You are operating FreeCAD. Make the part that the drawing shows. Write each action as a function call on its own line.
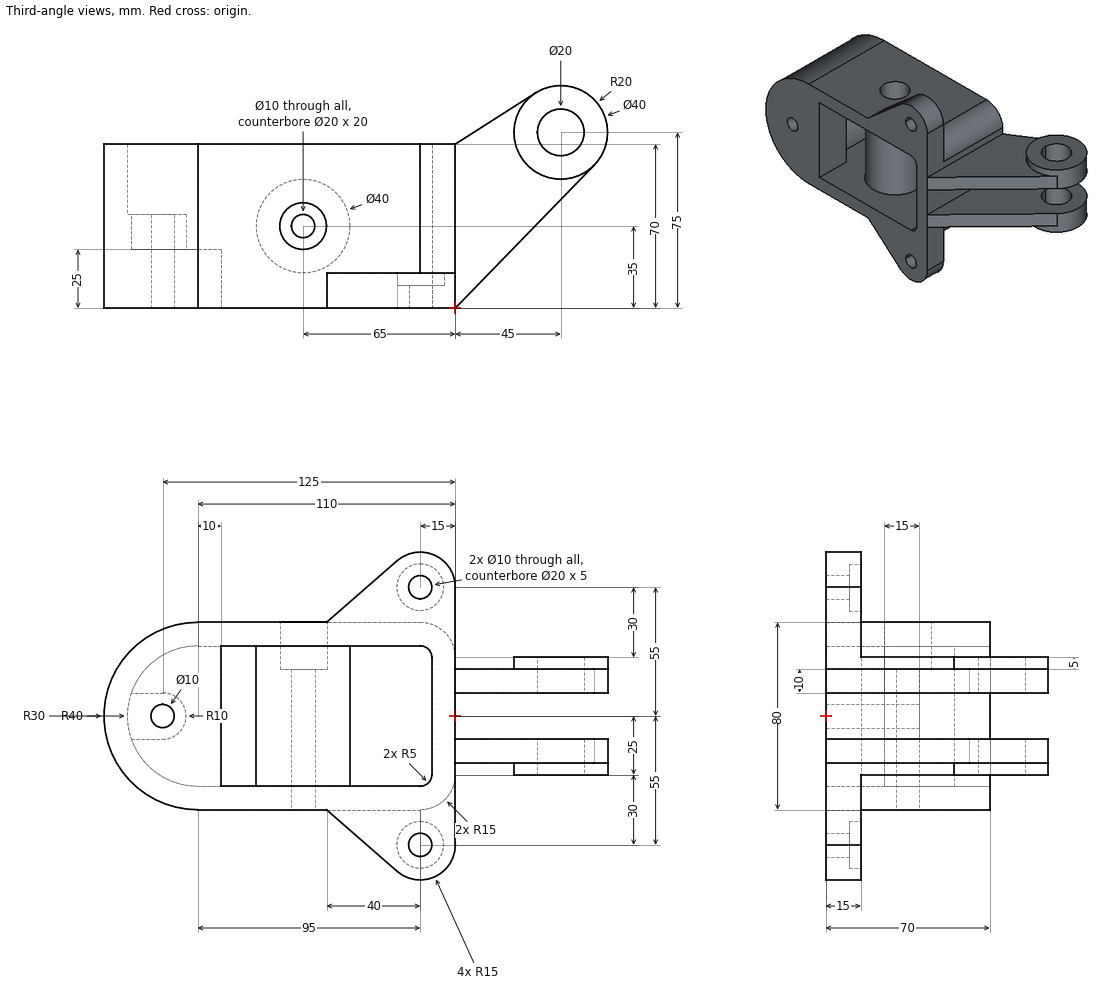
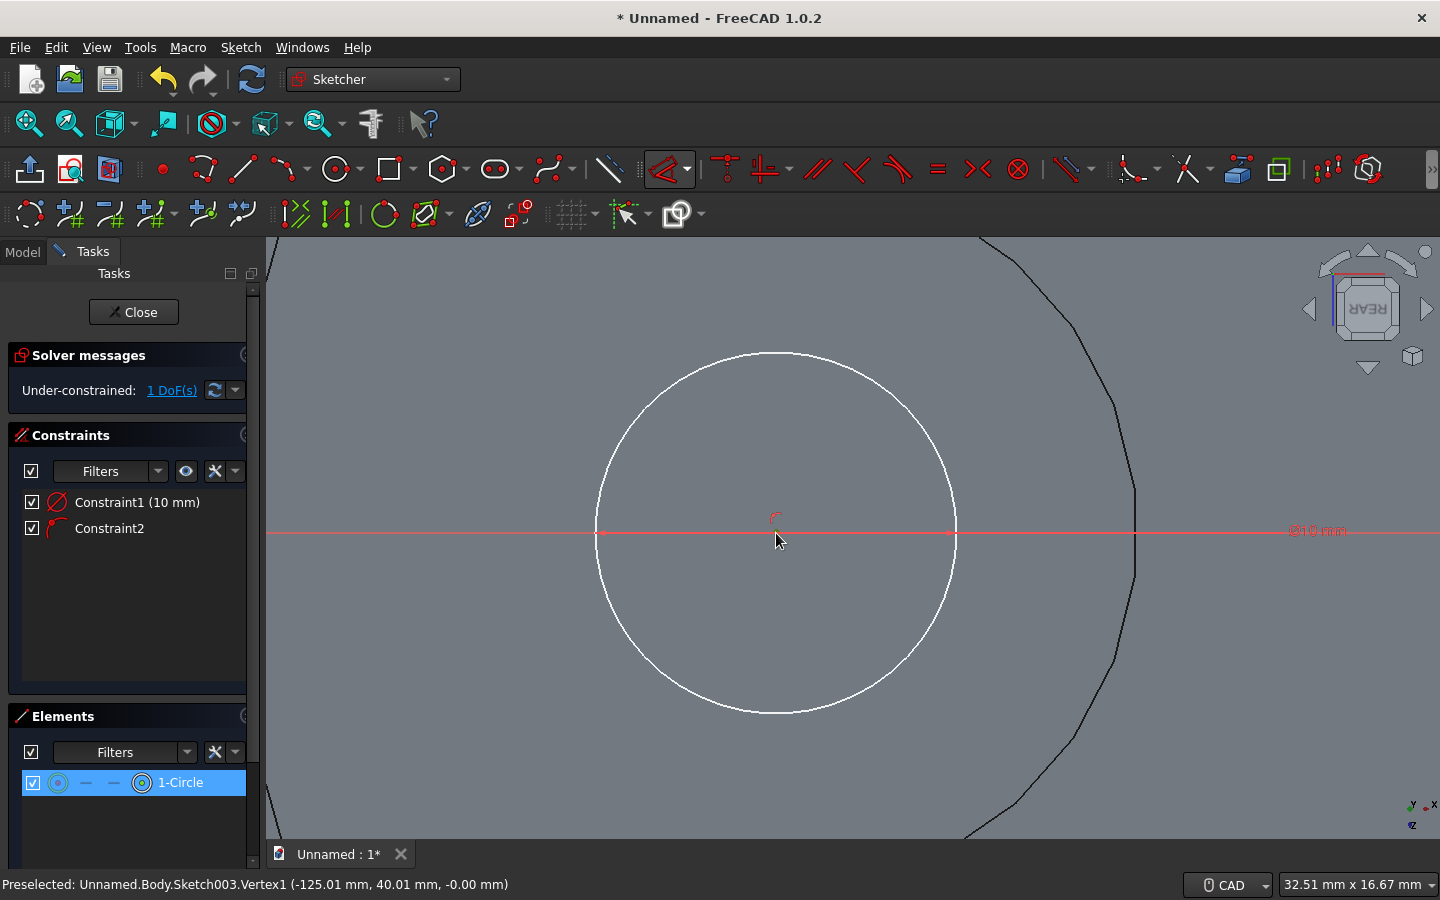
click(690, 170)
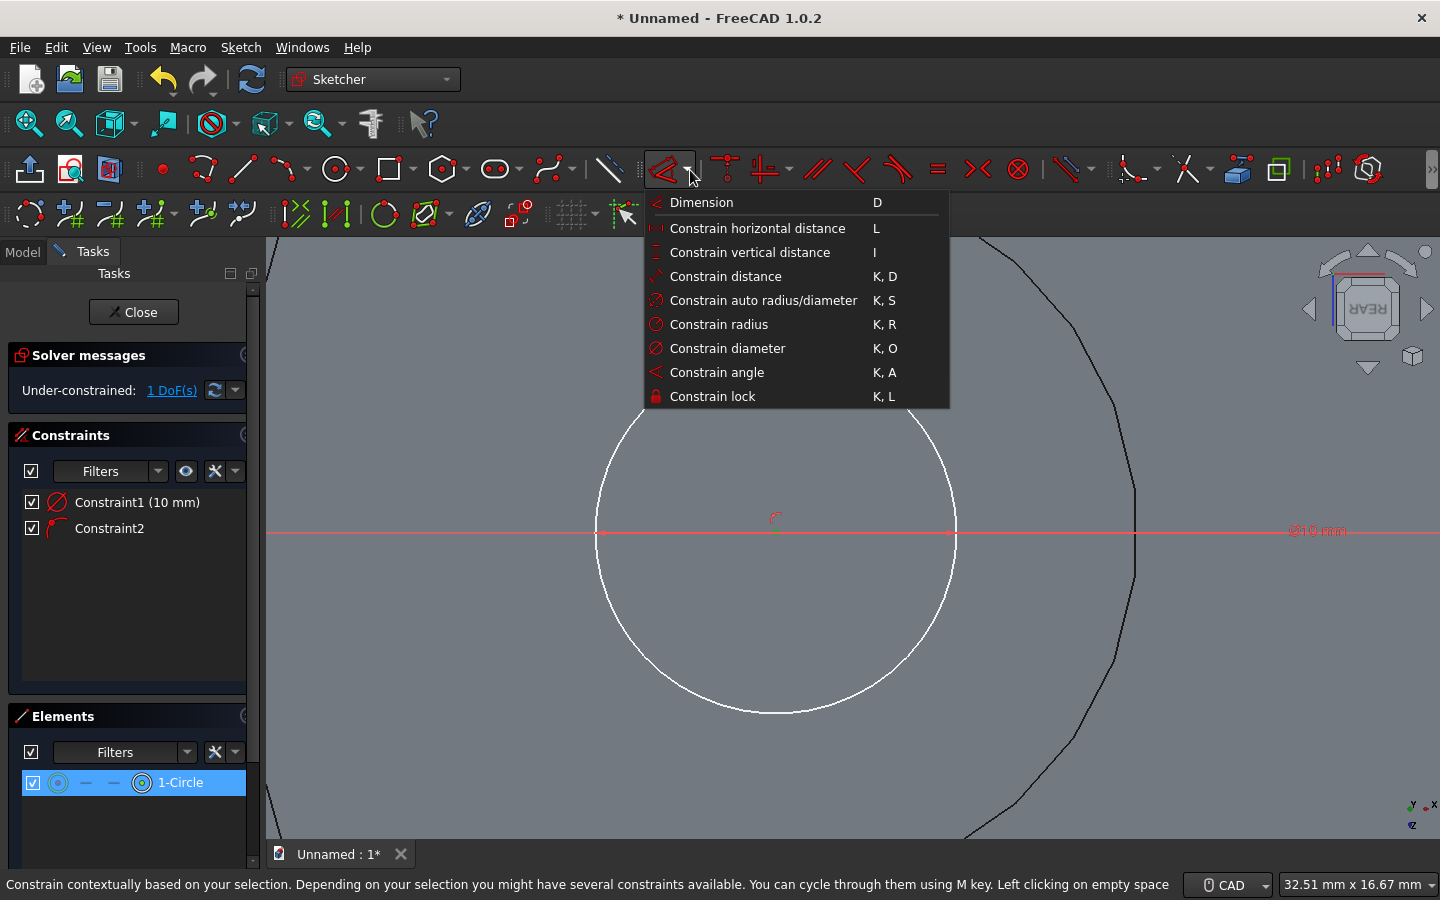
click(797, 228)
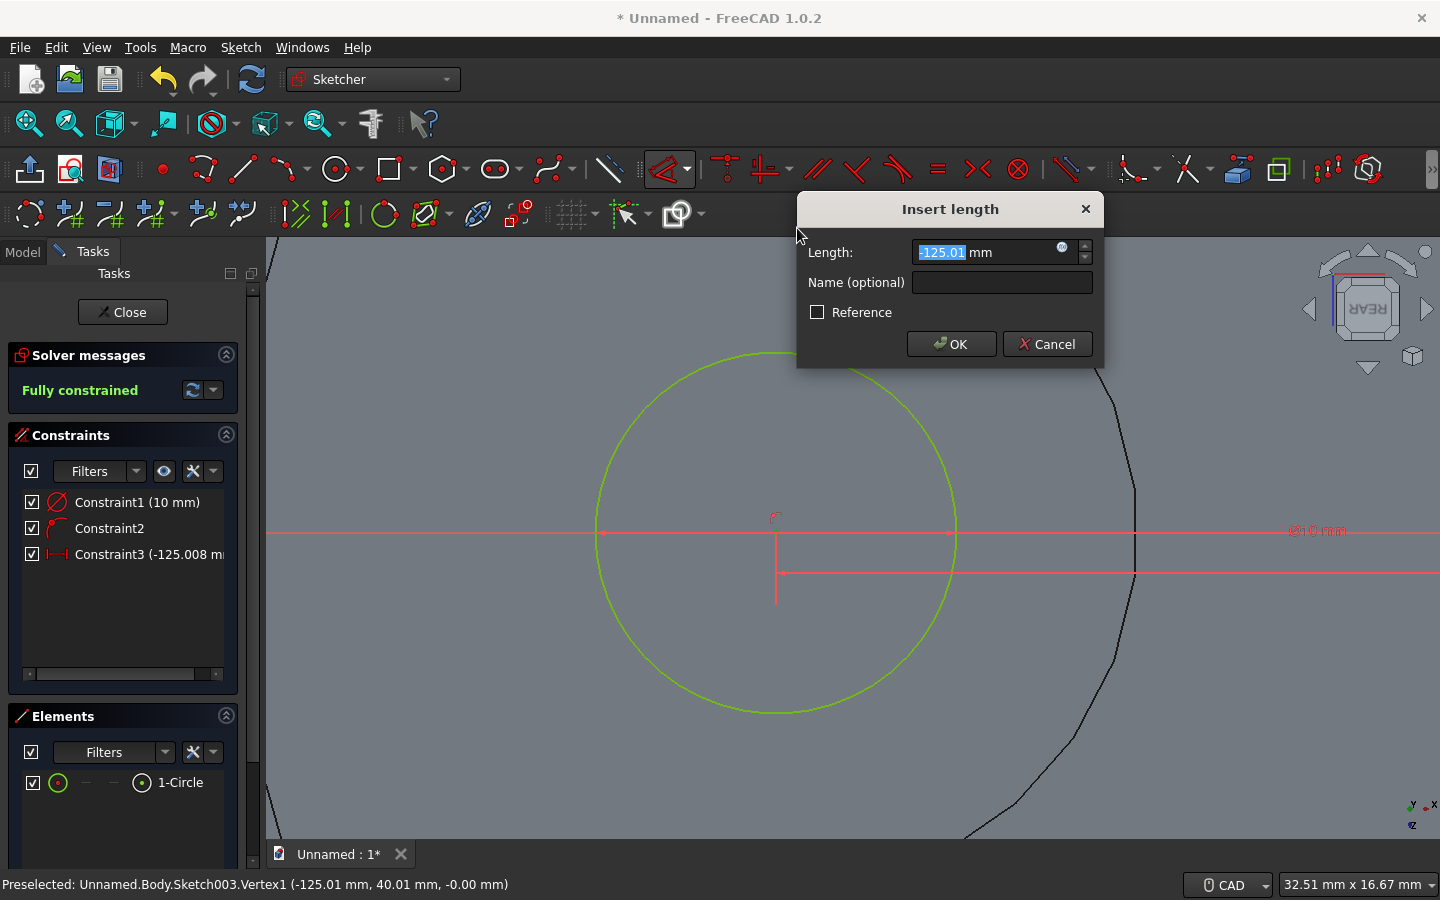
text(-125)
key(Return)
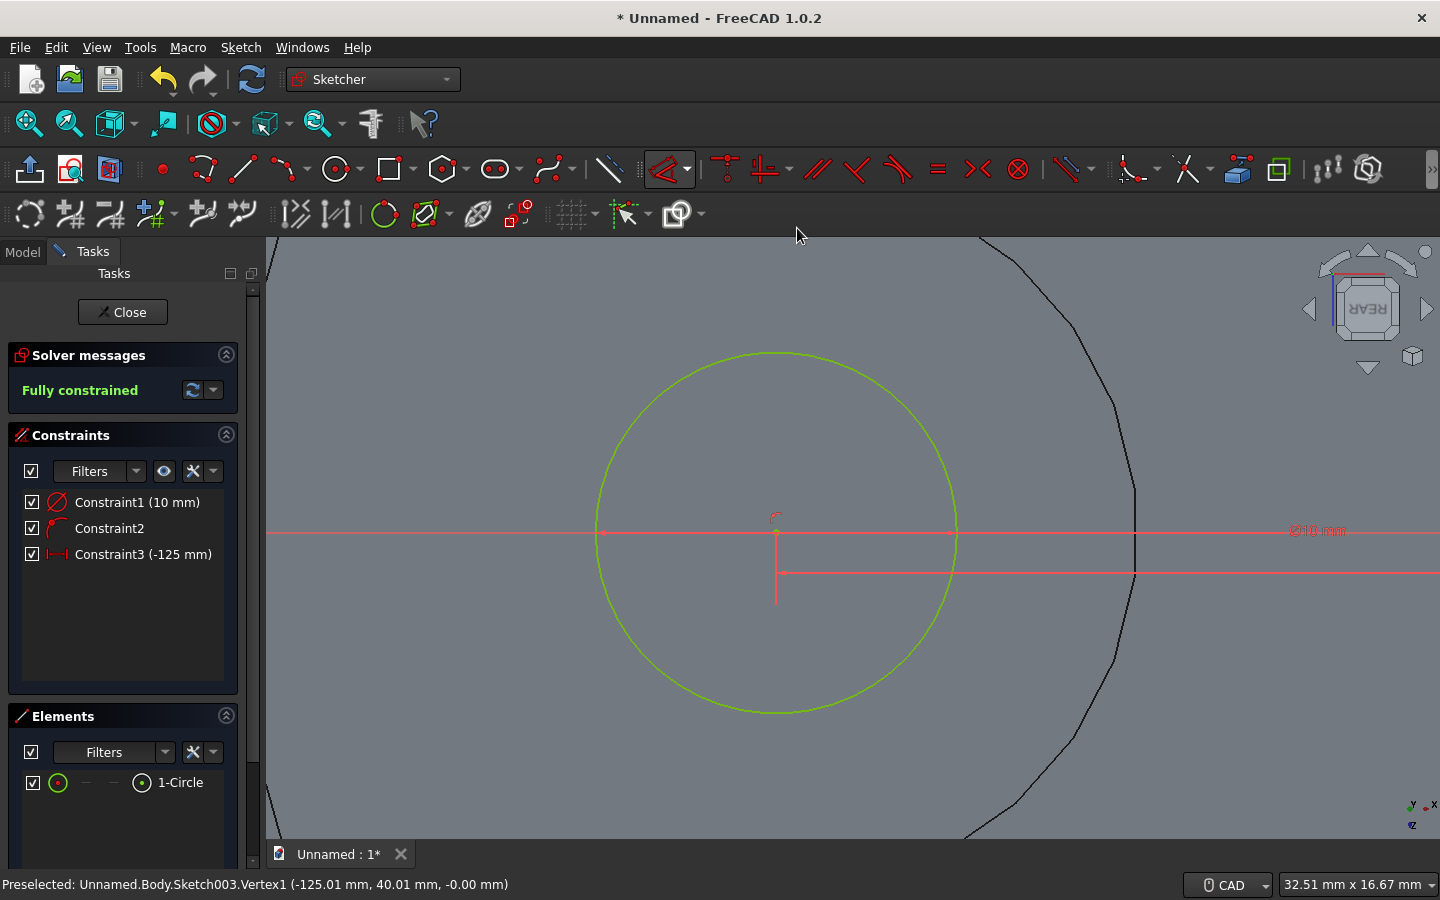
click(123, 312)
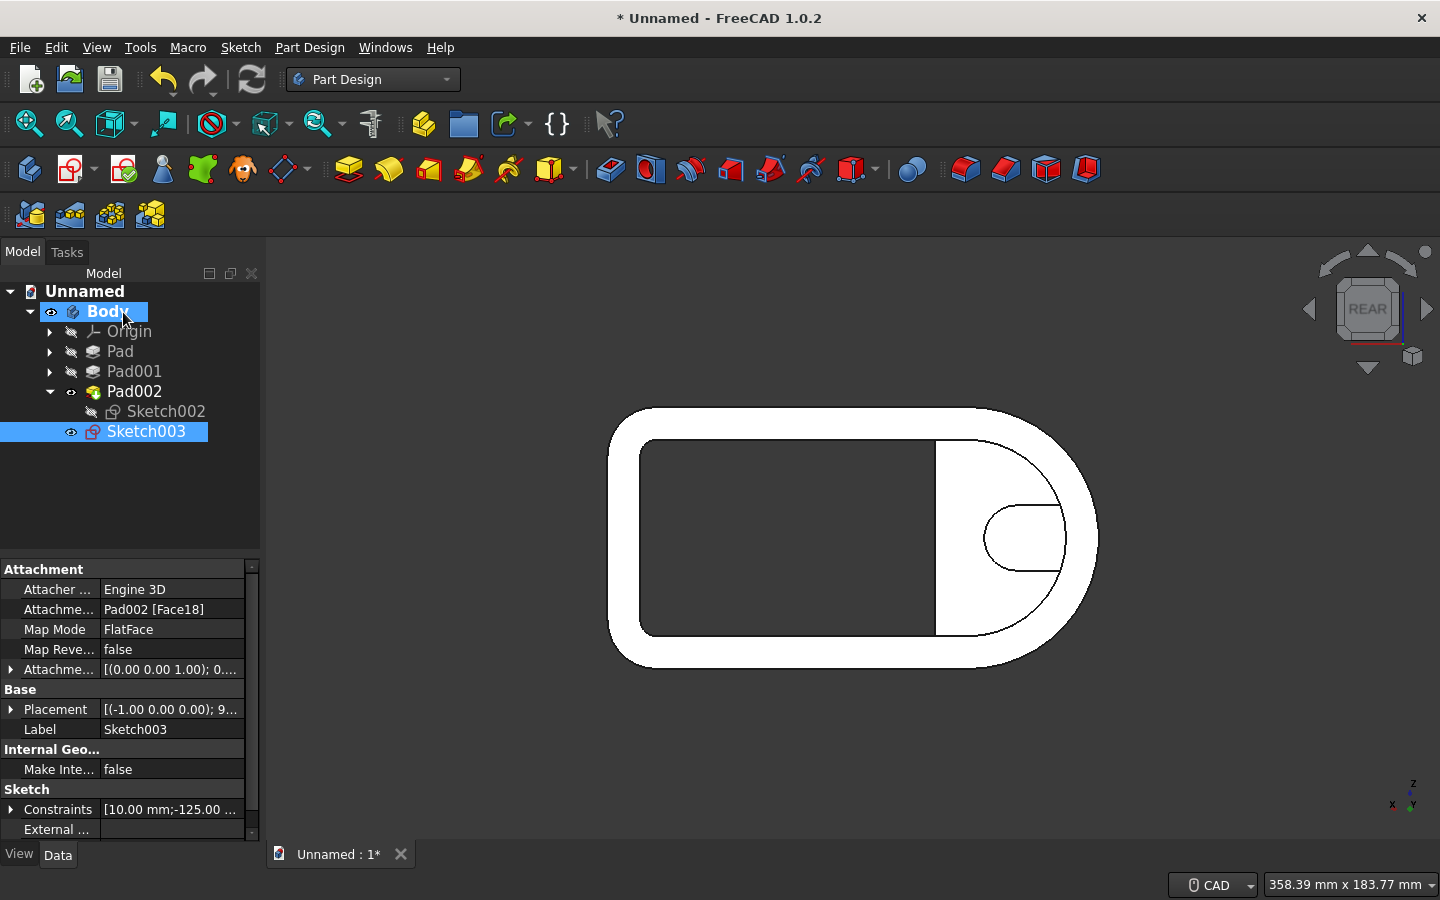
click(612, 170)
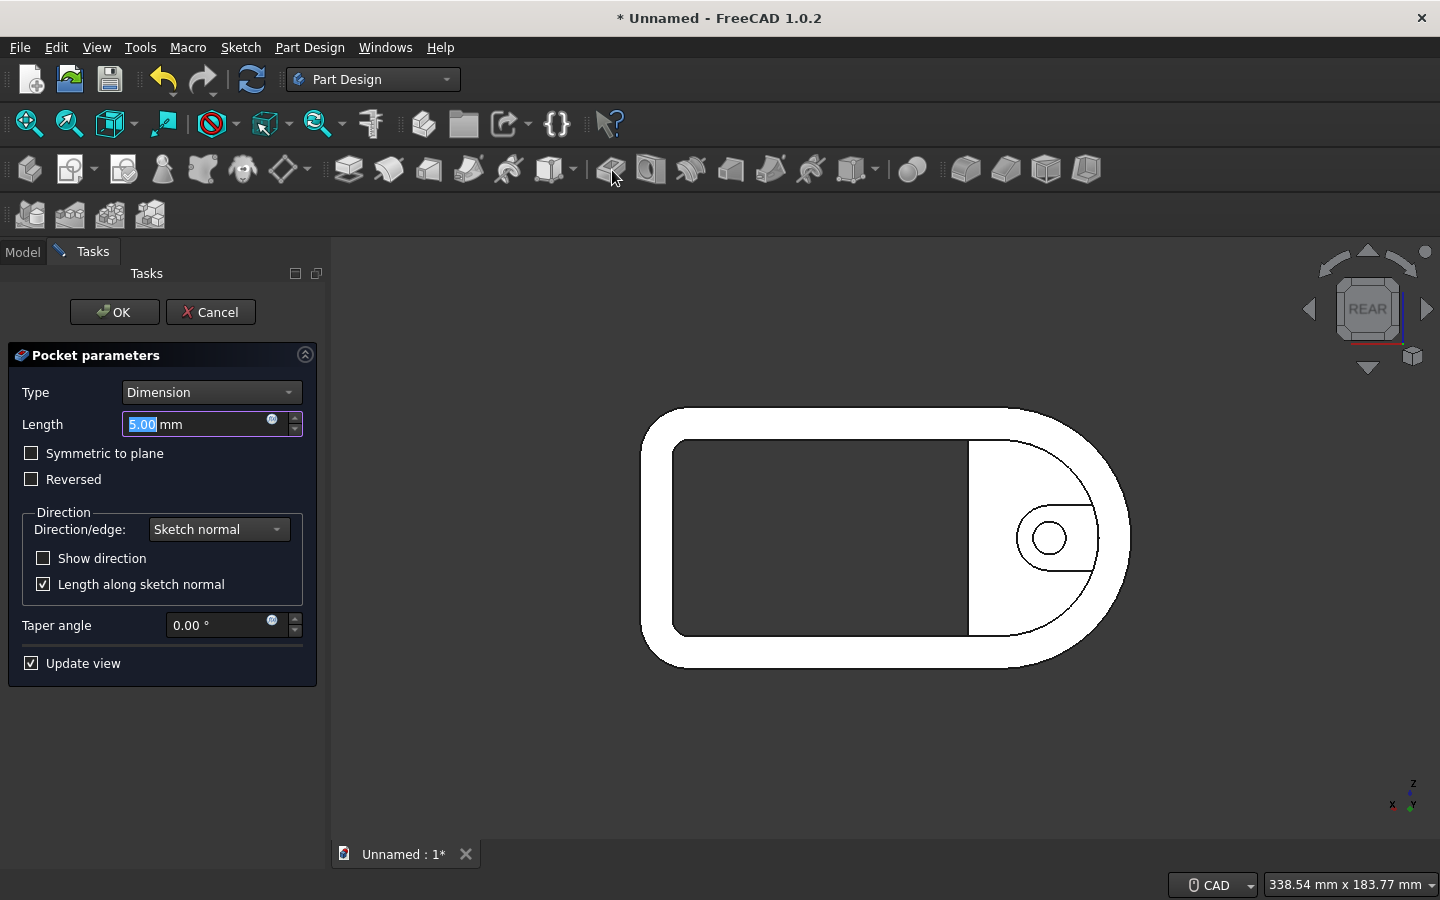
click(212, 392)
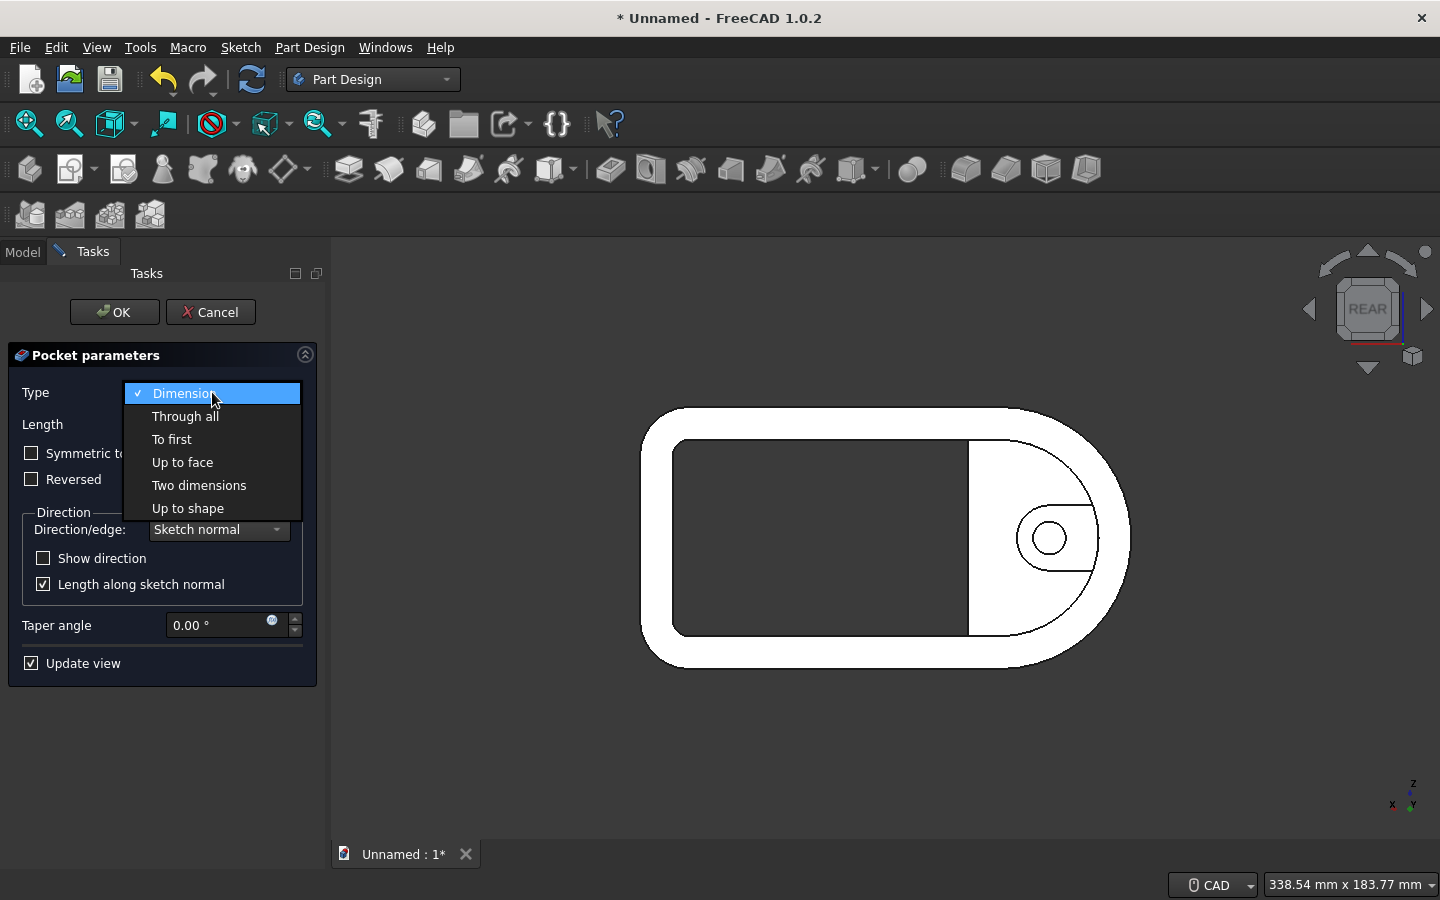
click(212, 416)